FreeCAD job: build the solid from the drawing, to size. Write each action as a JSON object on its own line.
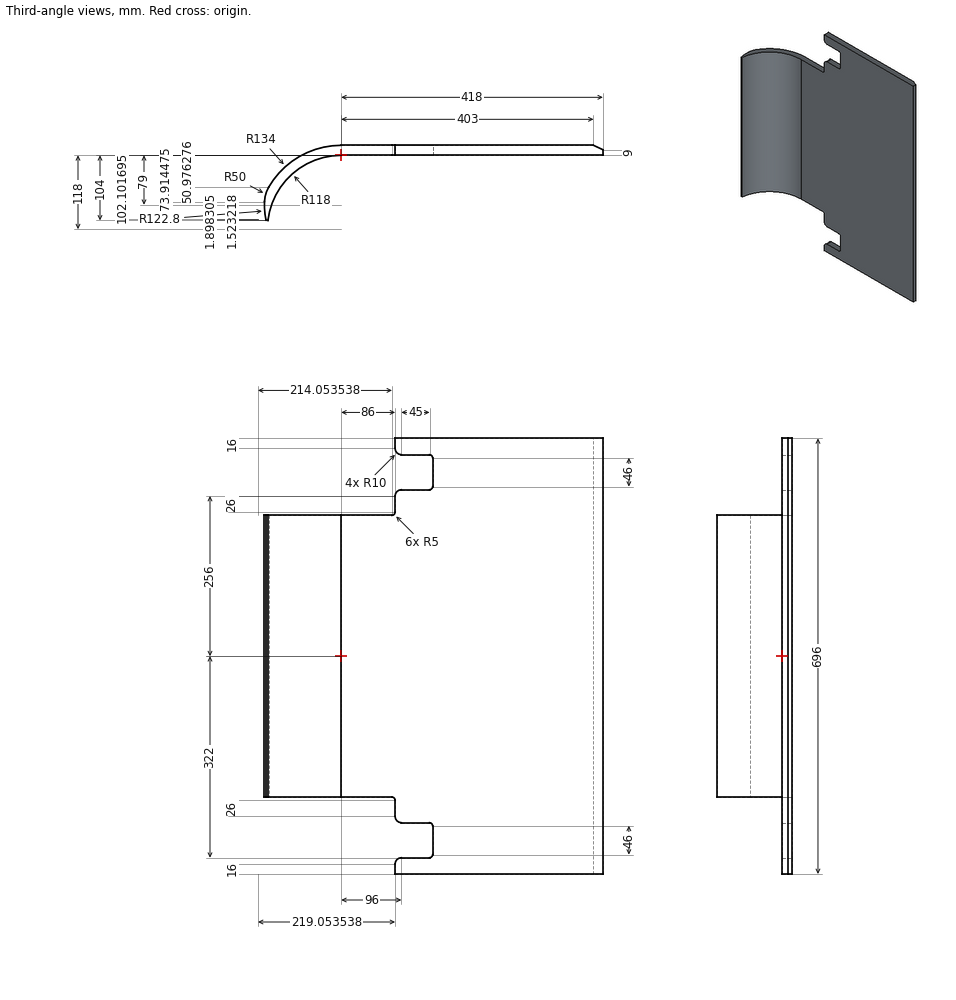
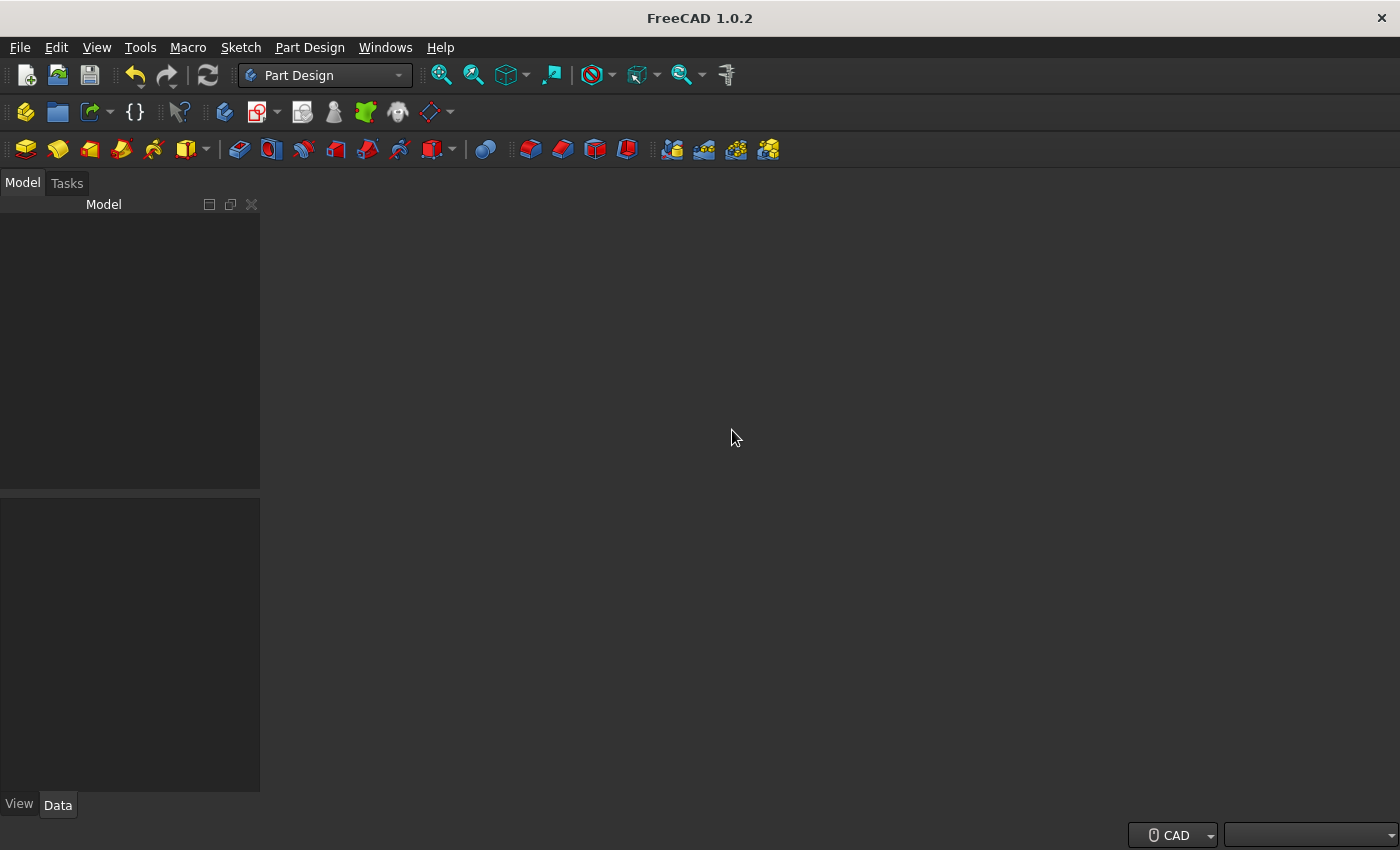
{"action": "left_click", "coordinate": [26, 76]}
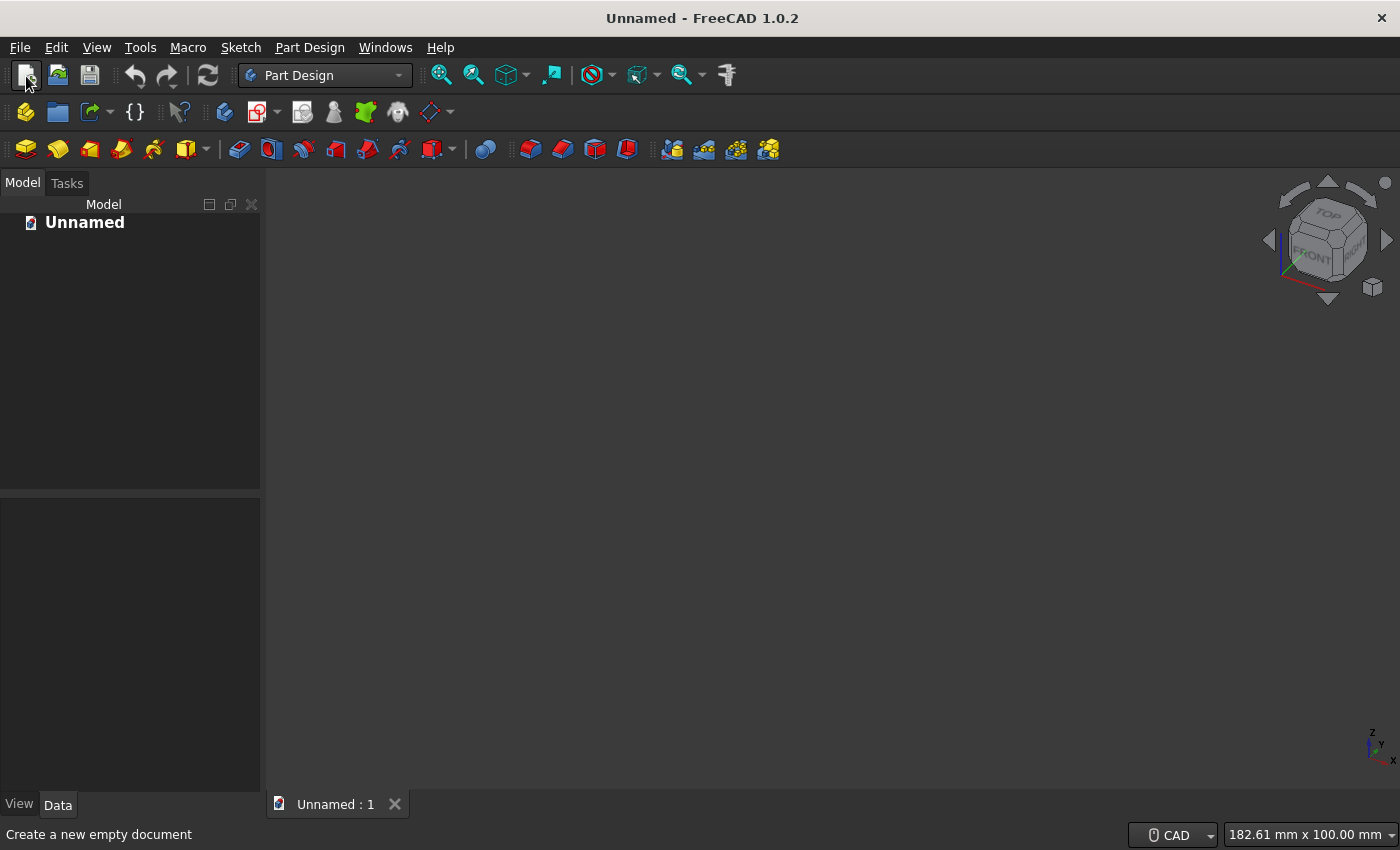
{"action": "left_click", "coordinate": [258, 112]}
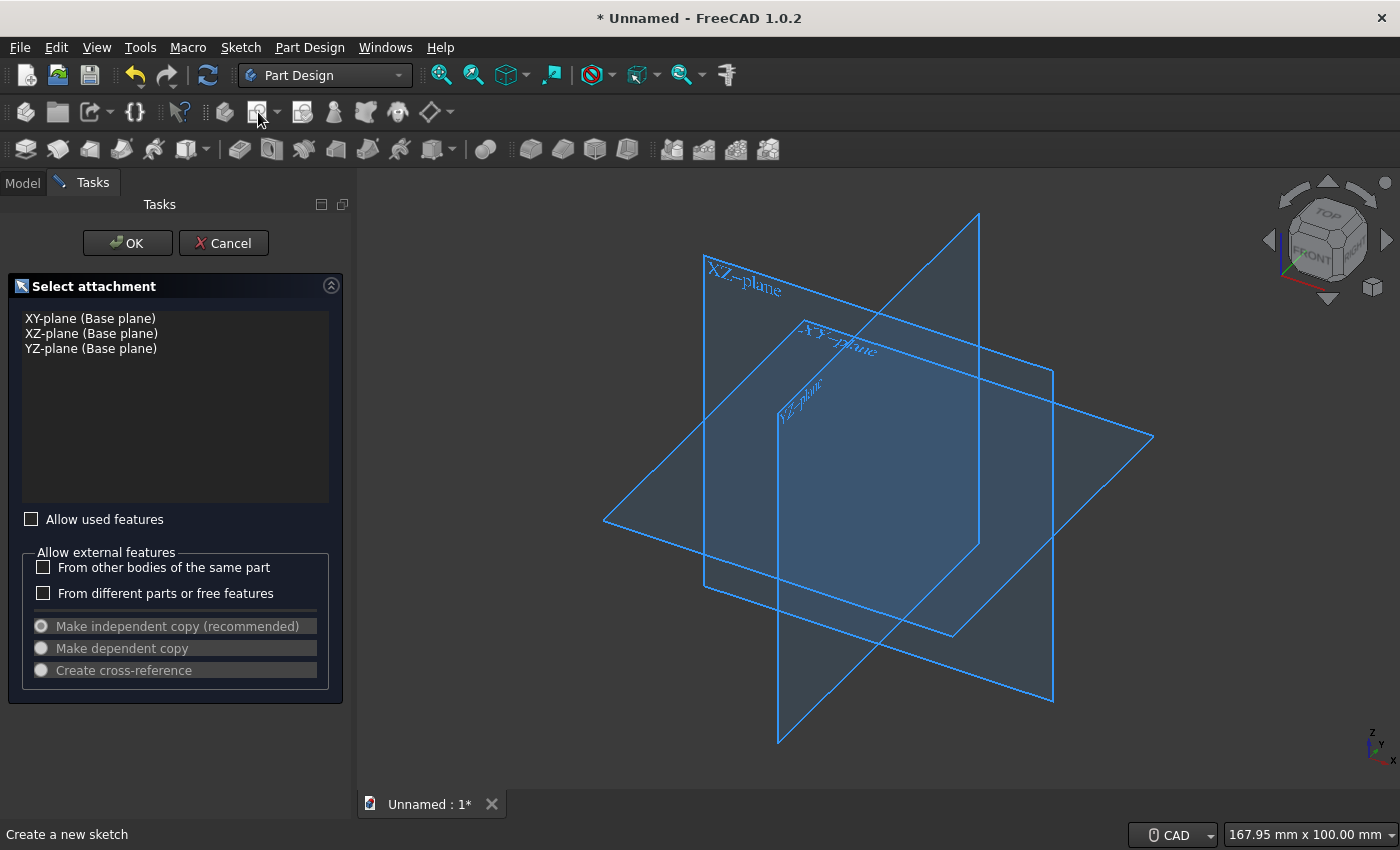
{"action": "left_click", "coordinate": [82, 318]}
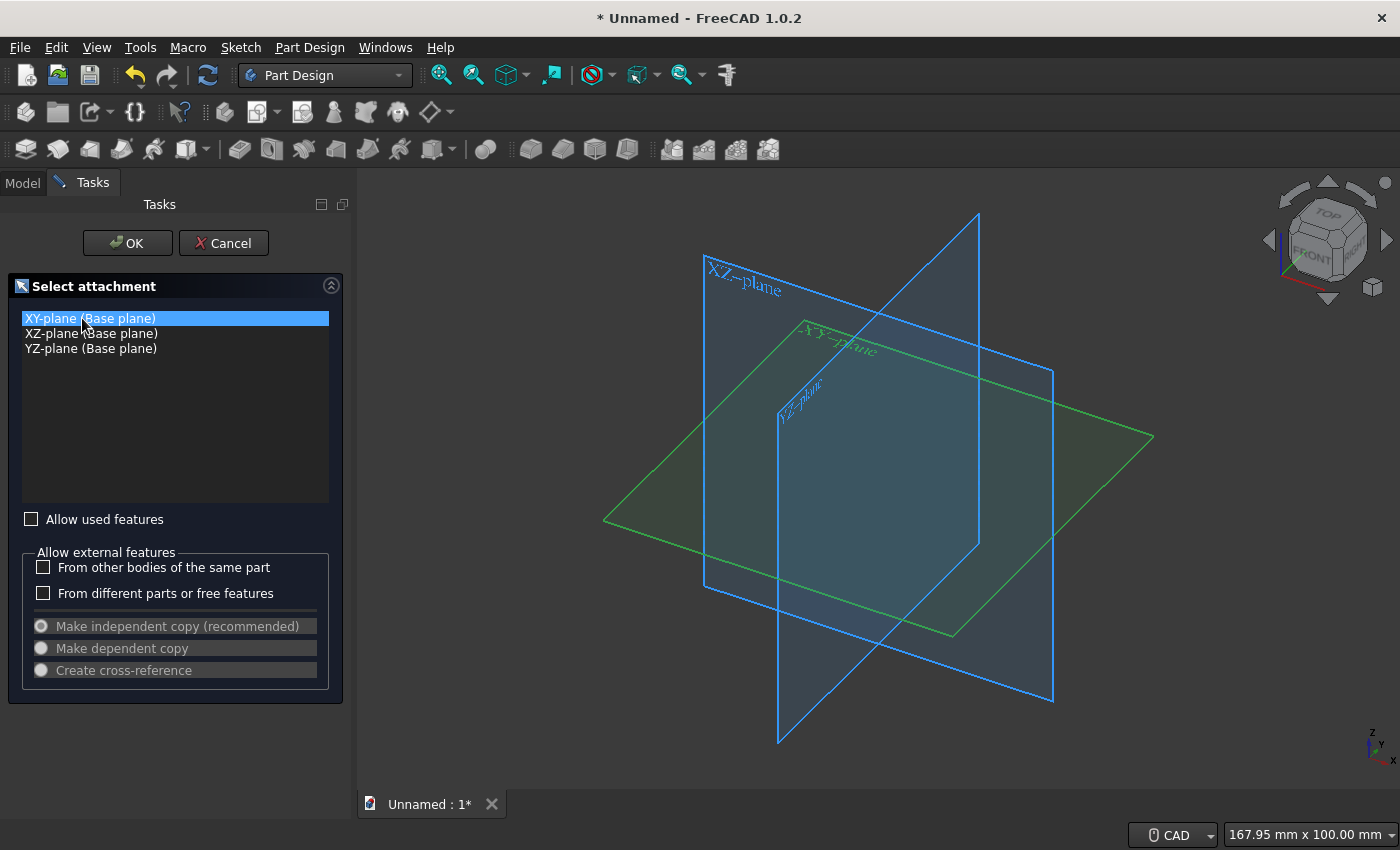
{"action": "left_click", "coordinate": [128, 243]}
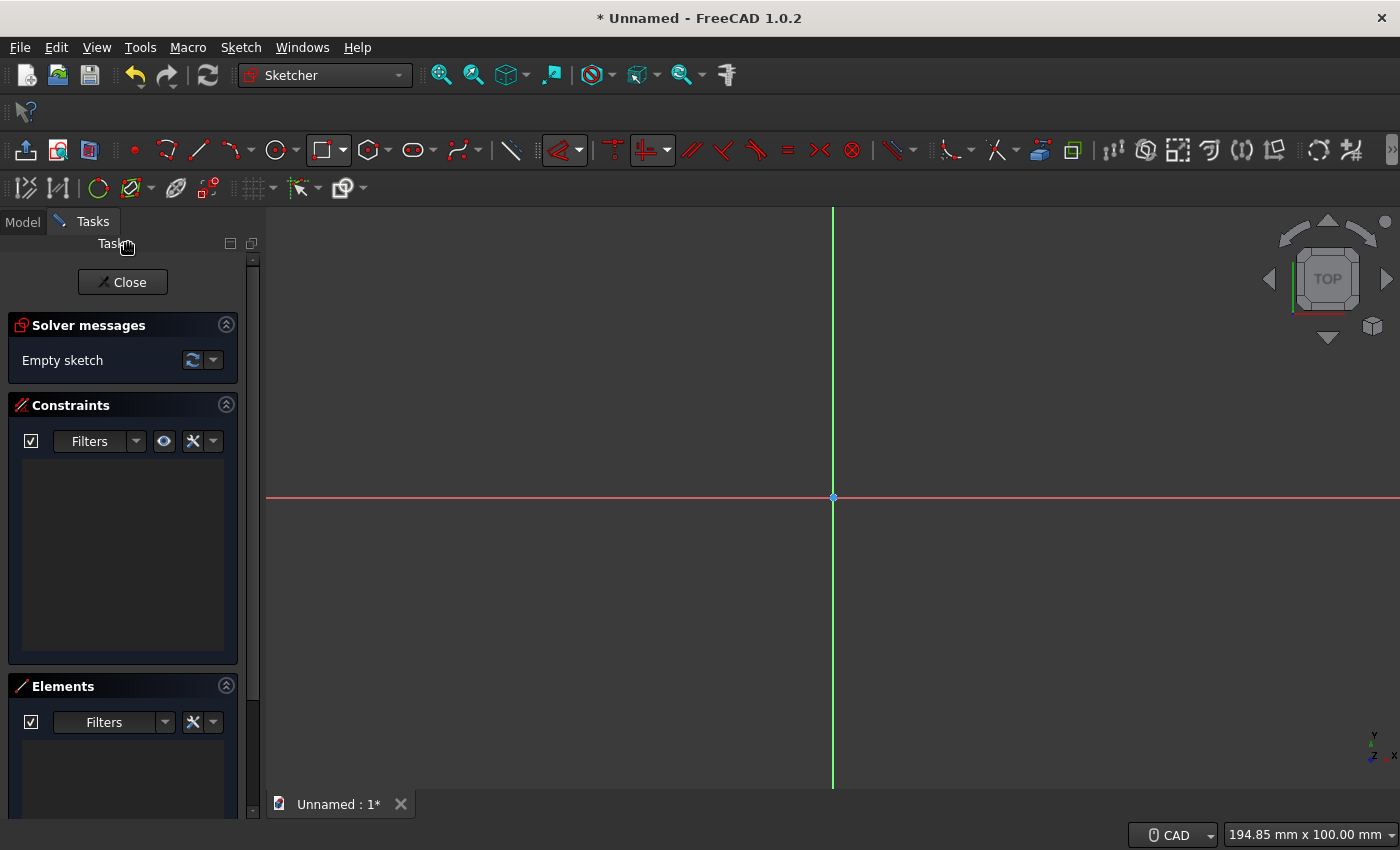
{"action": "scroll", "coordinate": [537, 433], "scroll_direction": "down", "scroll_amount": 8}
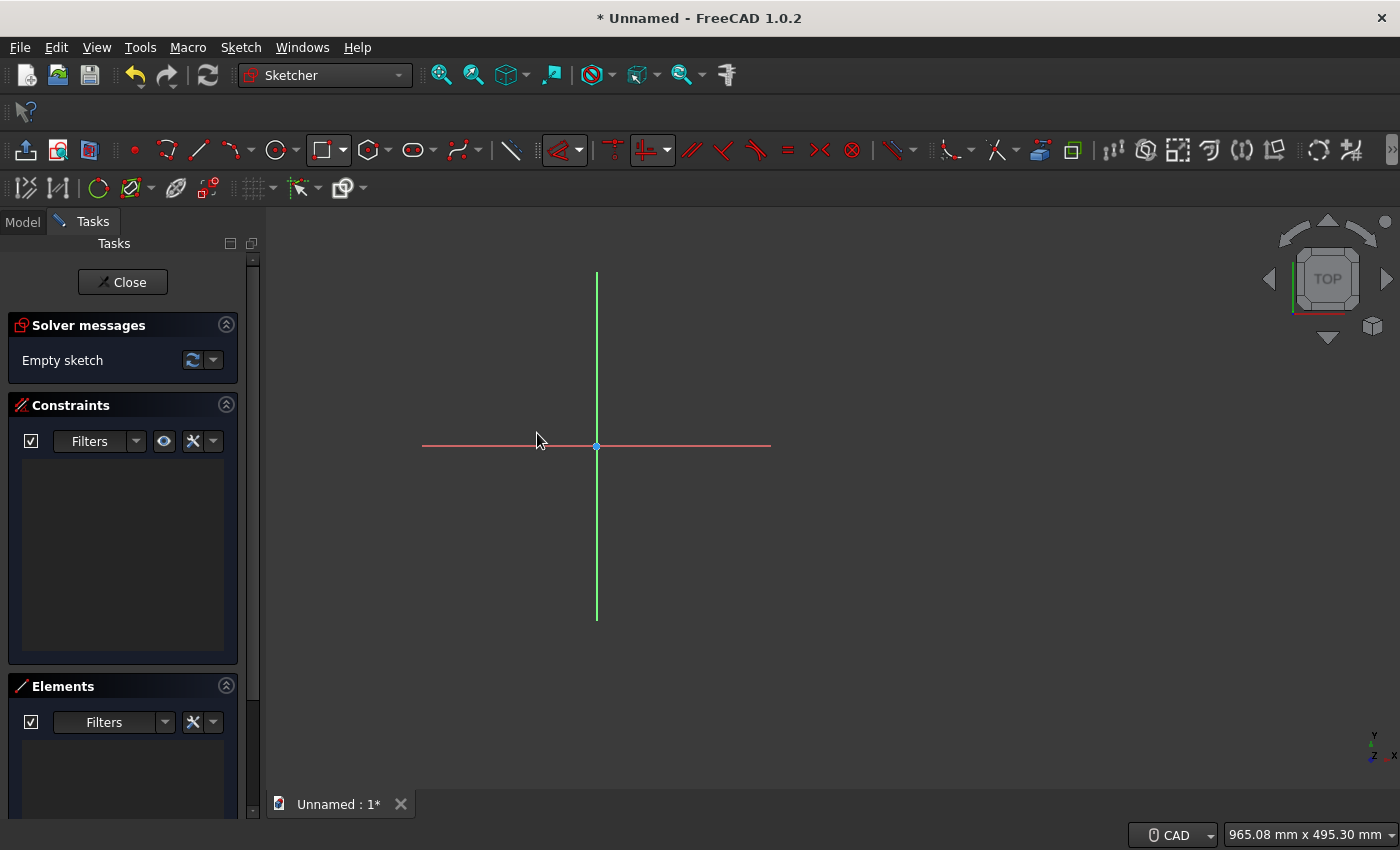
{"action": "left_click", "coordinate": [168, 150]}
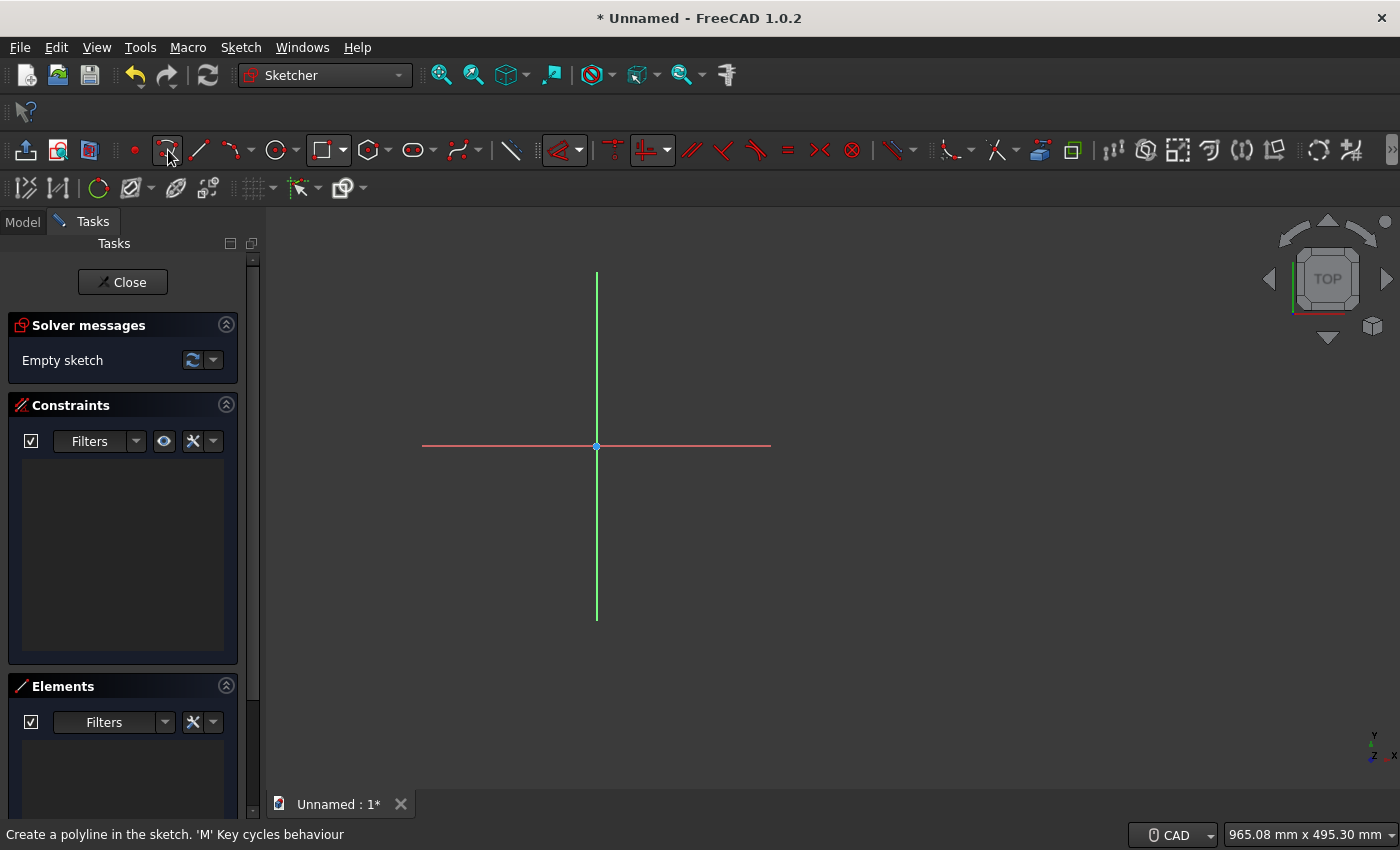
{"action": "left_click", "coordinate": [597, 446]}
{"action": "left_click", "coordinate": [1088, 455]}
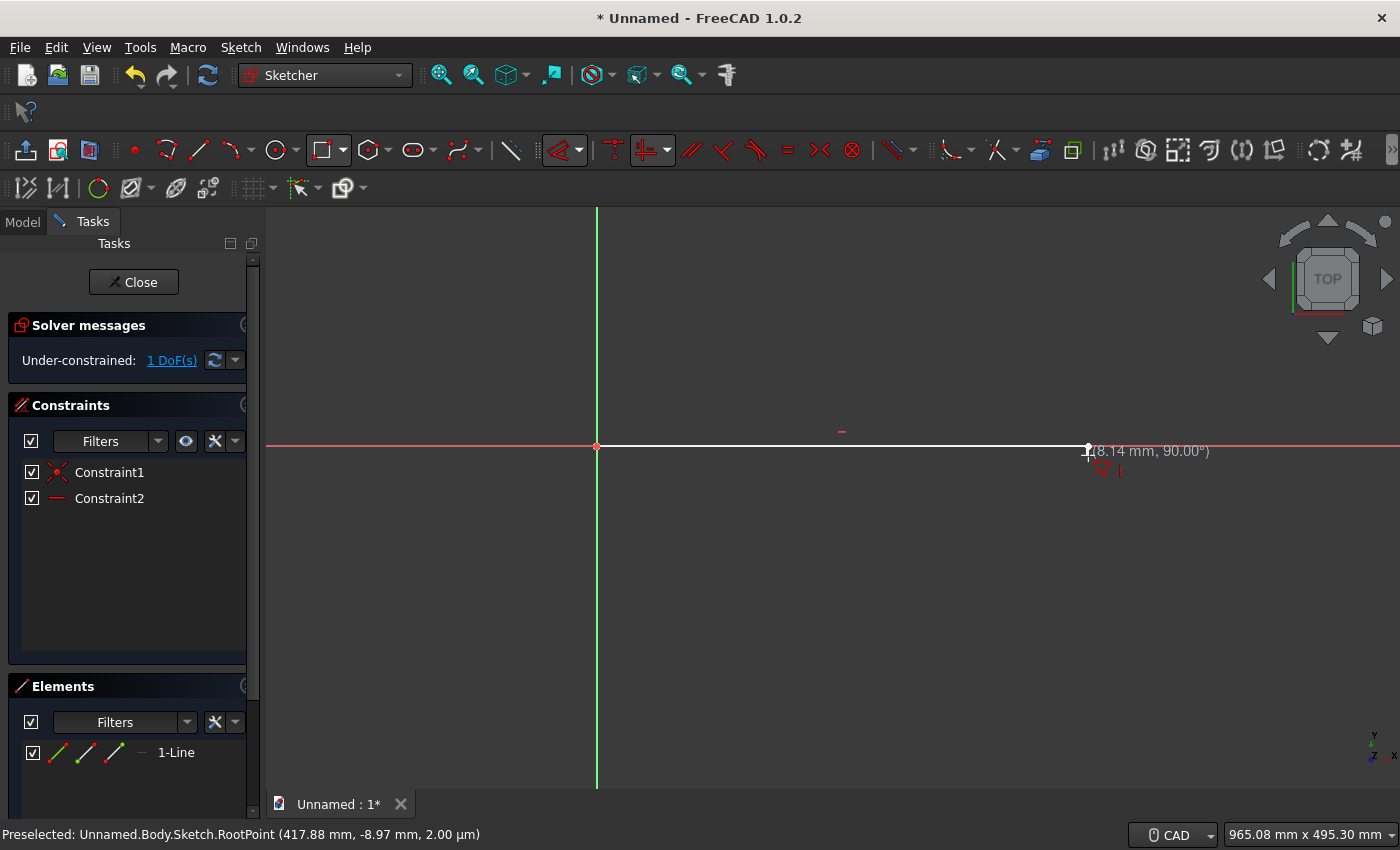
{"action": "scroll", "coordinate": [1088, 436], "scroll_direction": "up", "scroll_amount": 3}